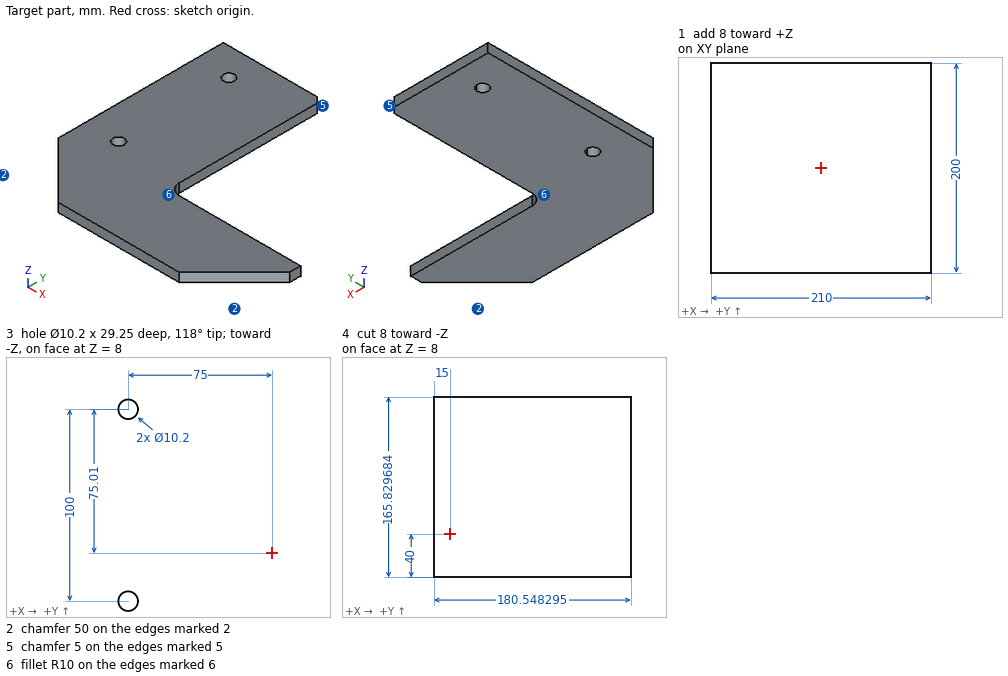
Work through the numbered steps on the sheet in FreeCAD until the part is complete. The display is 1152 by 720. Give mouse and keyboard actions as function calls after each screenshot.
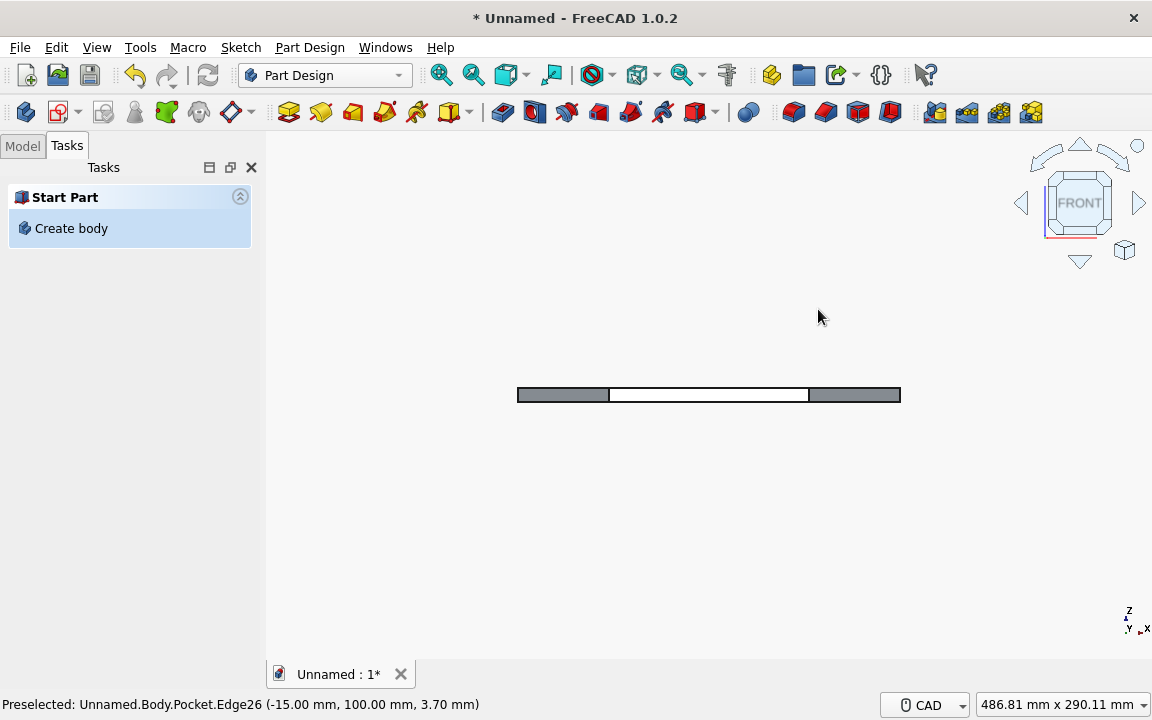
scroll(682, 394, up, 6)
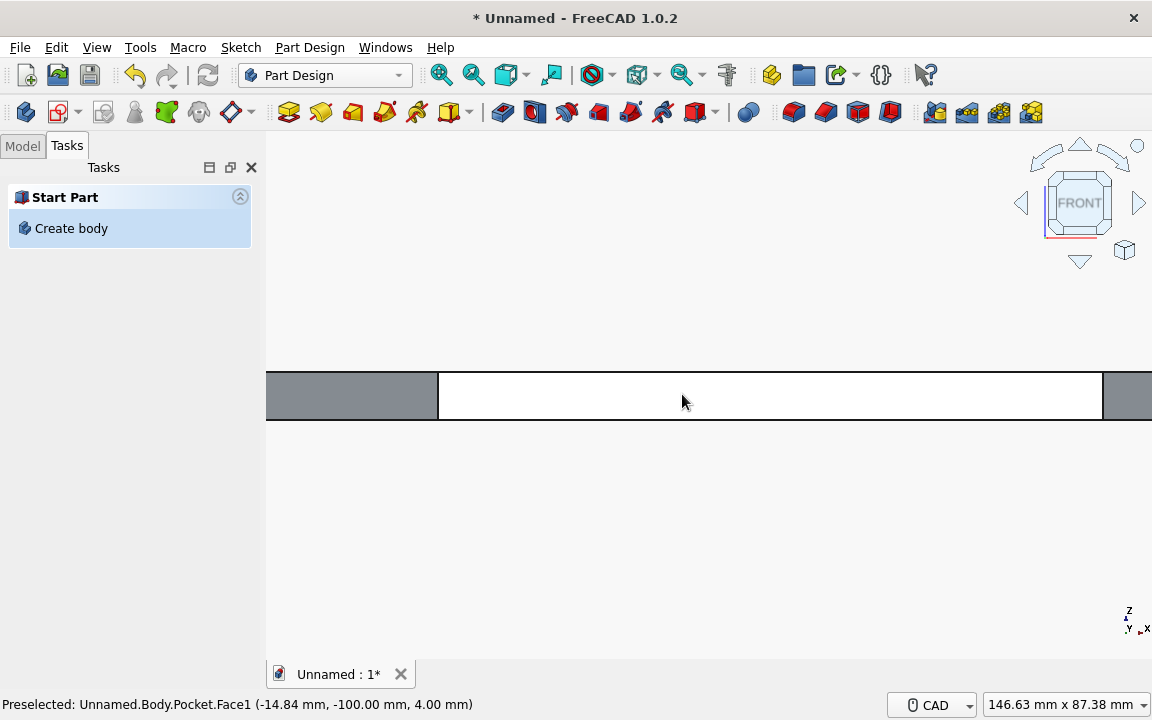
key(v)
key(f)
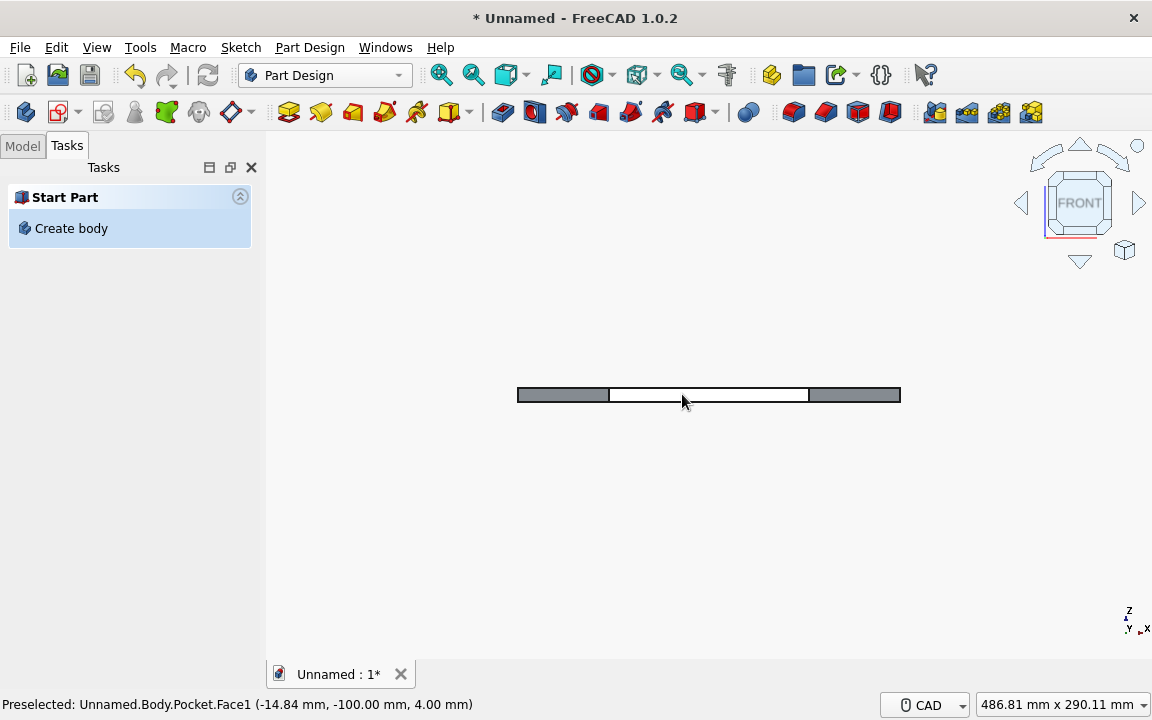
key(3)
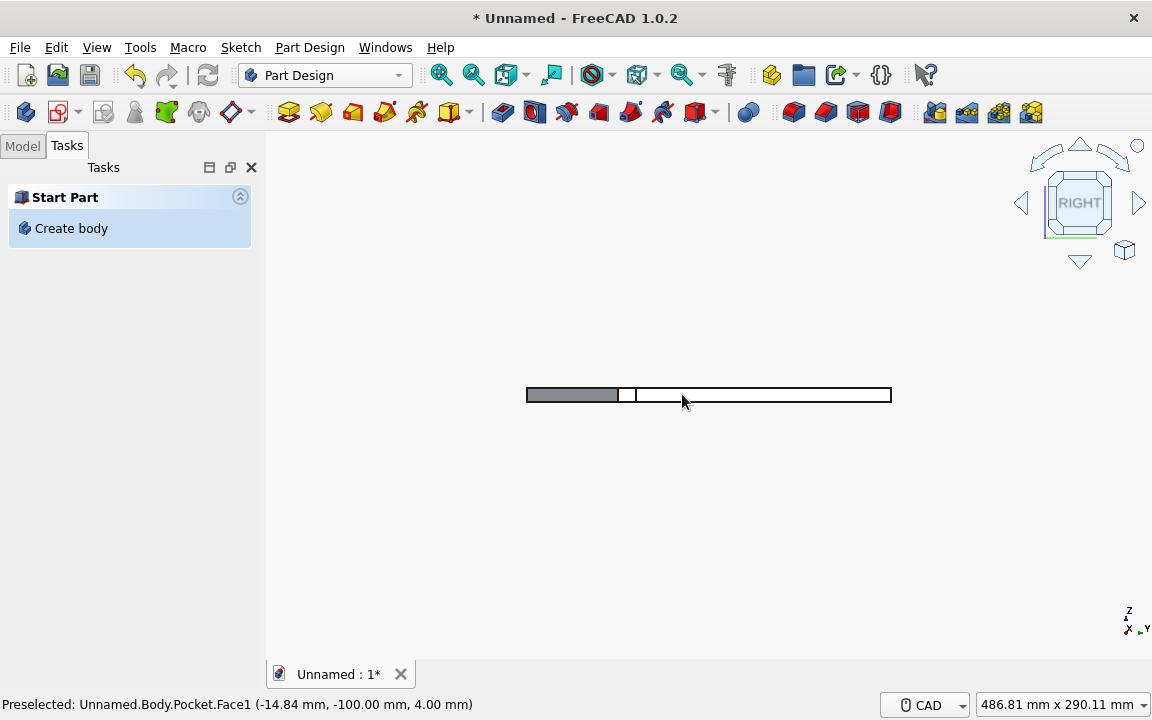
click(442, 76)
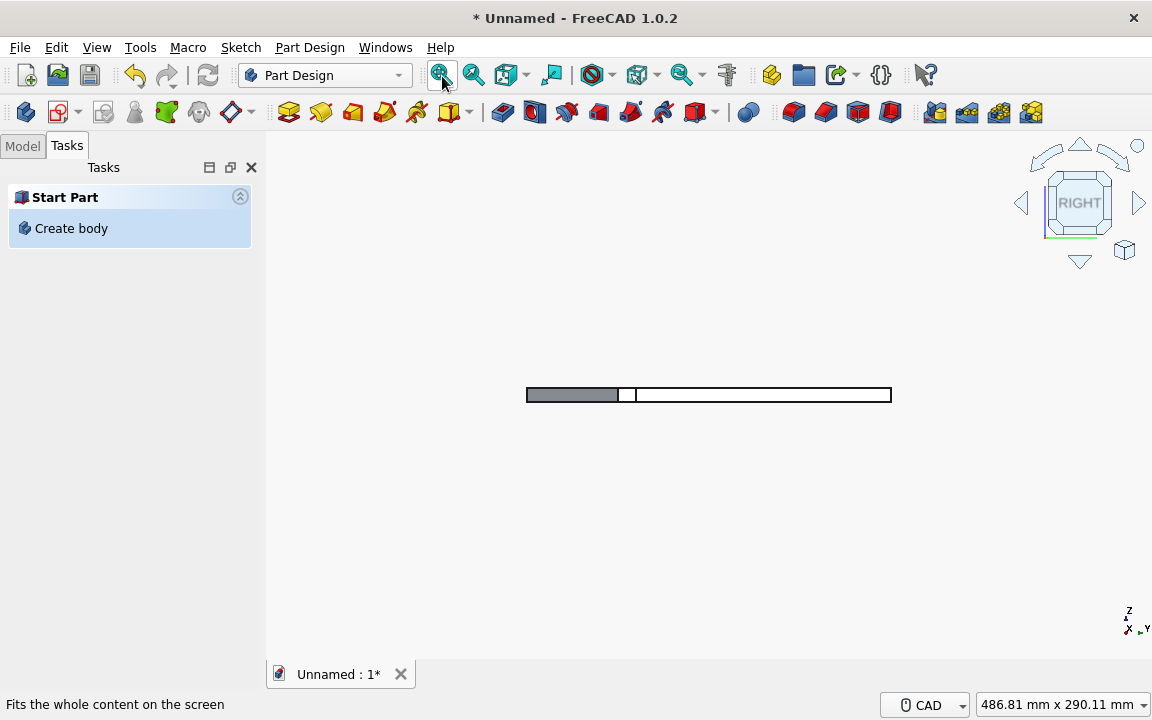
click(891, 394)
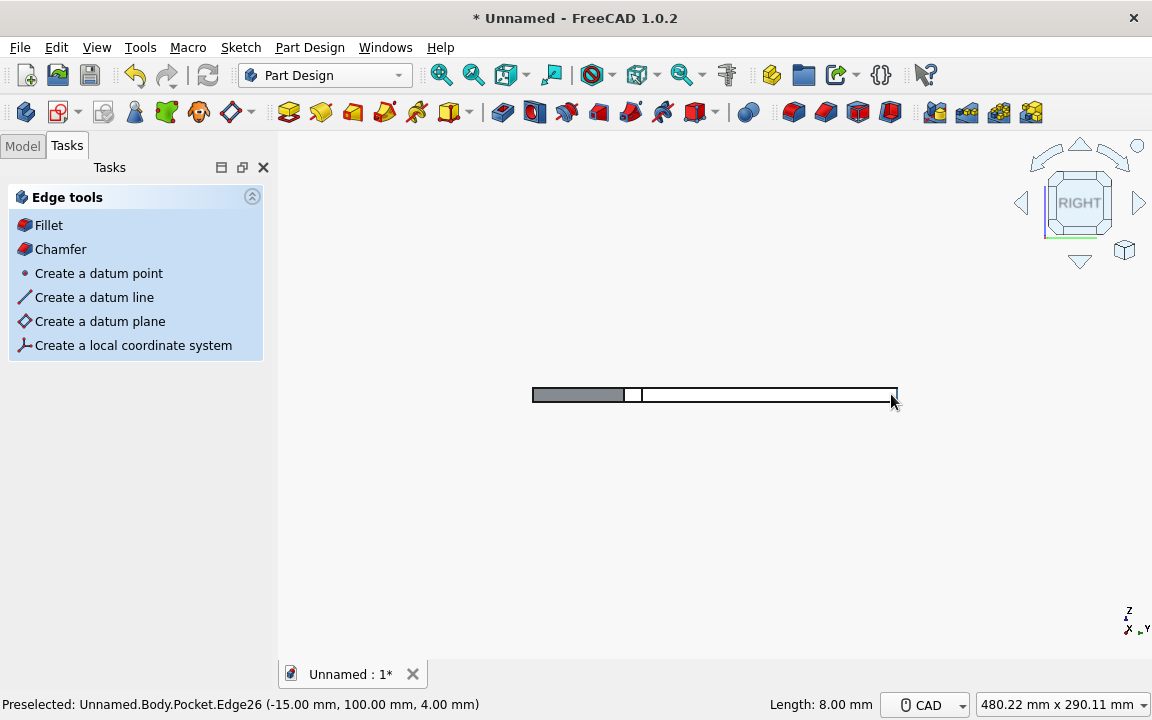
click(826, 112)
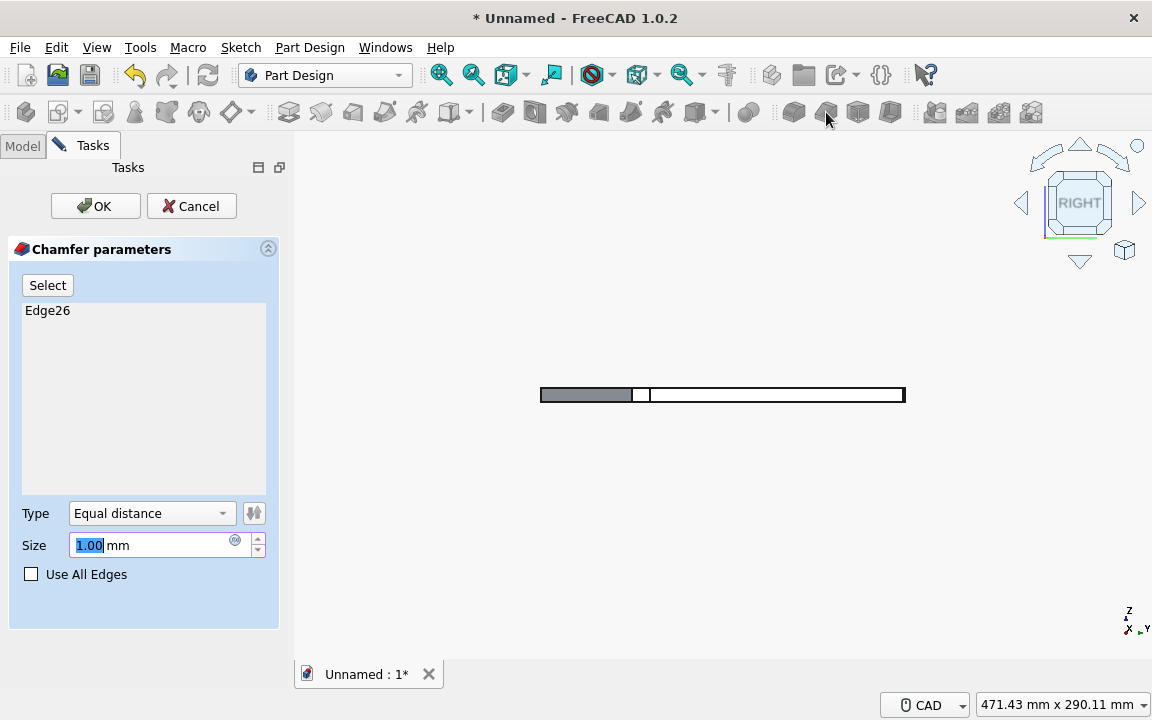
text(5)
key(Tab)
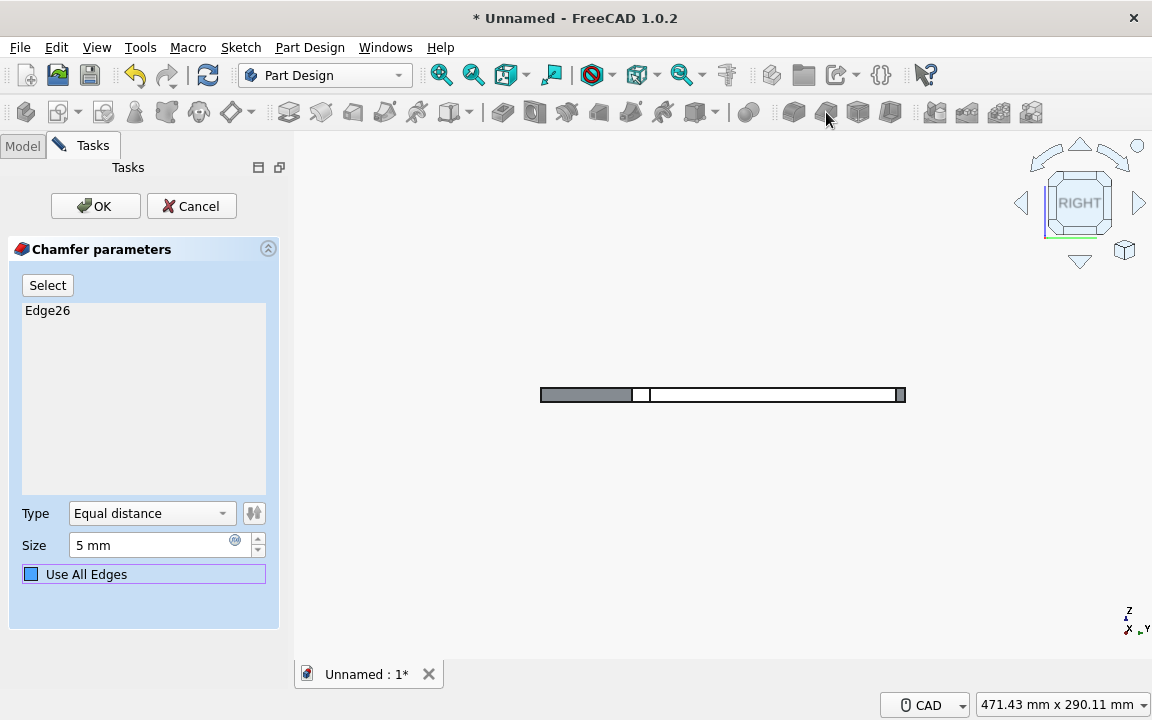
click(96, 206)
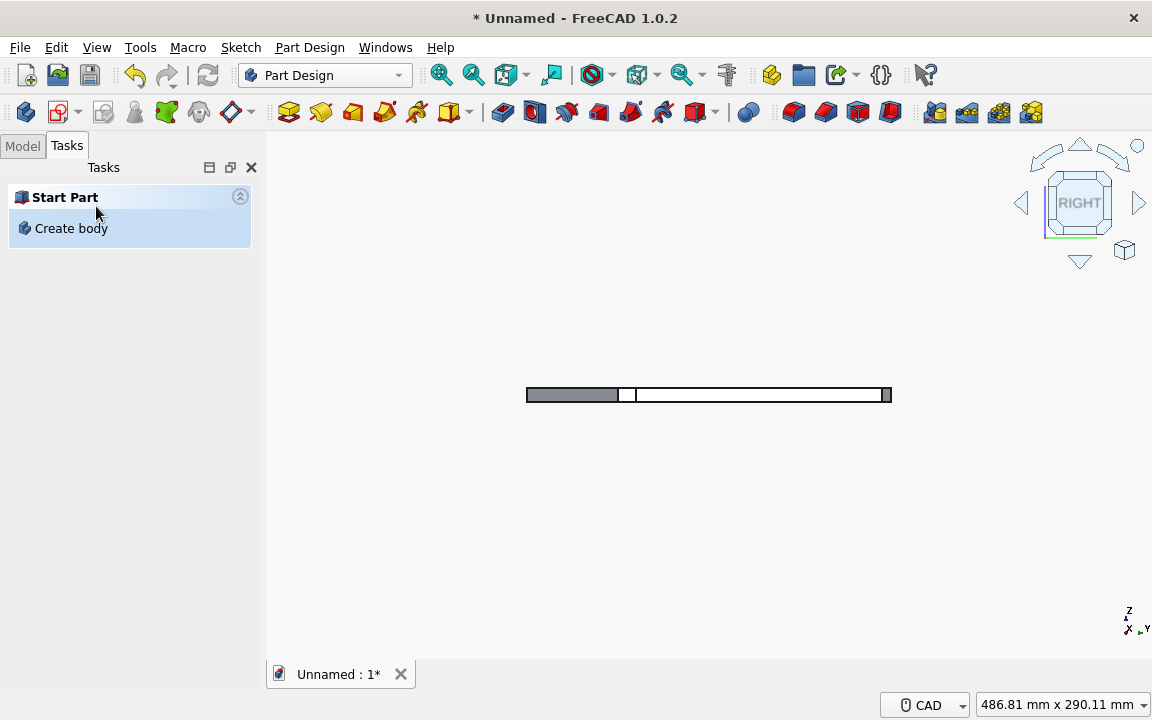
click(442, 76)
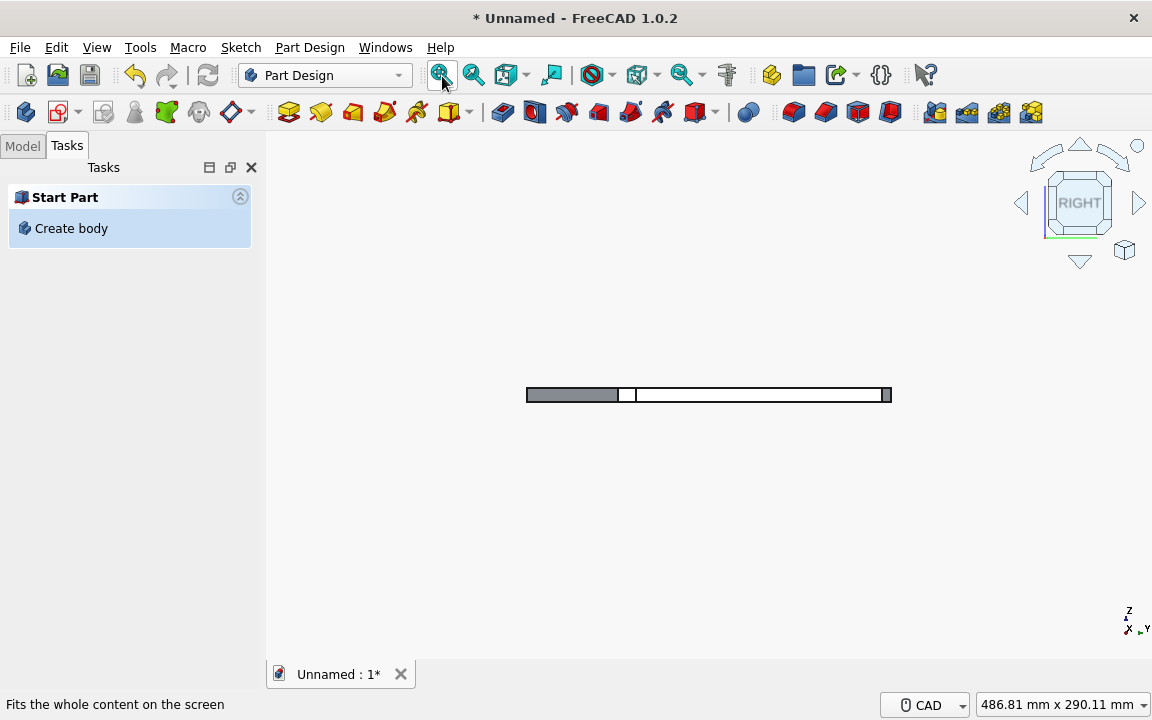
scroll(636, 394, up, 6)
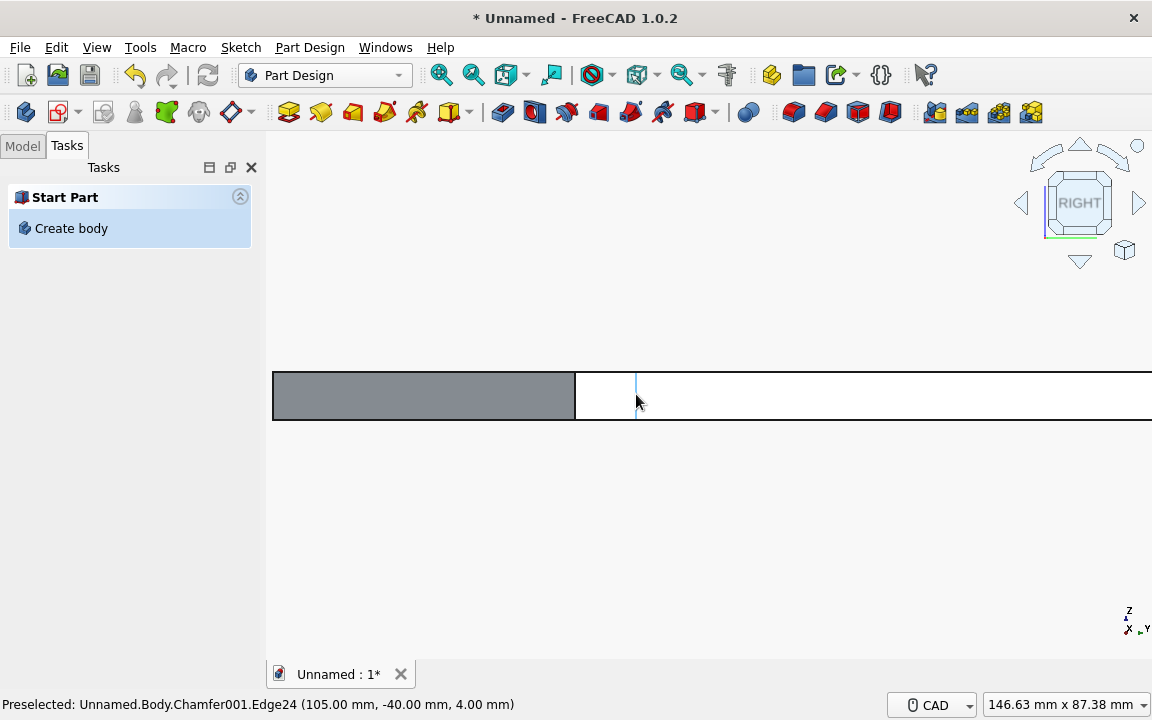
key(v)
key(f)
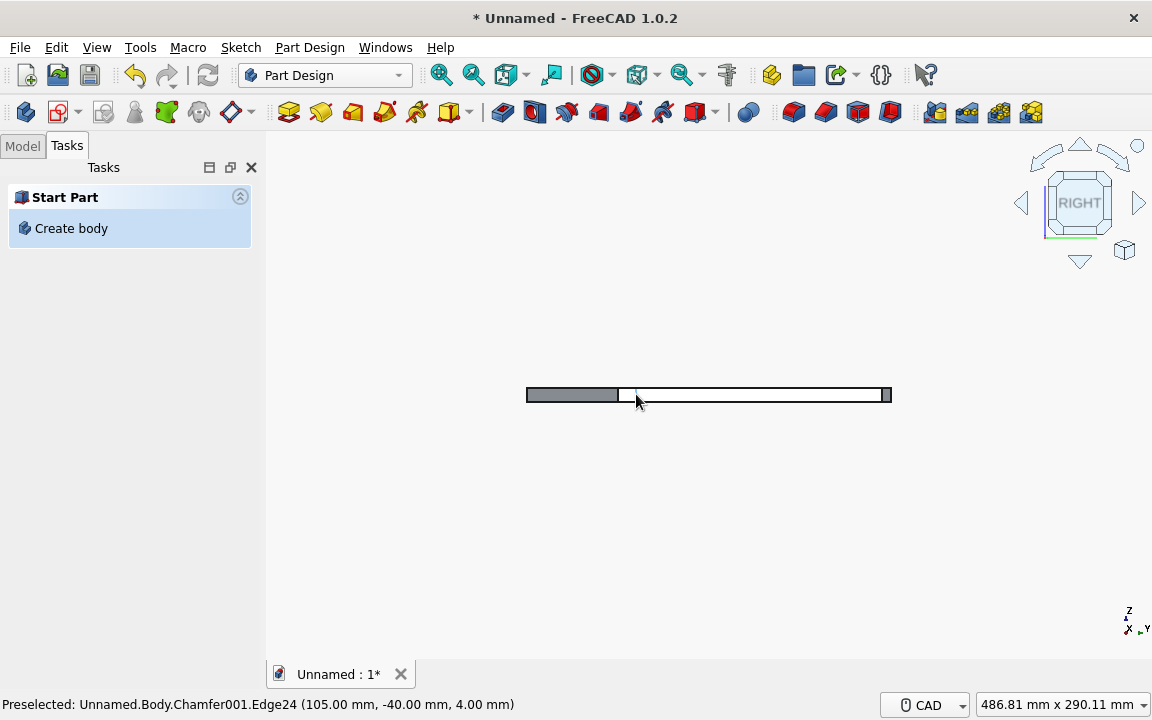
key(0)